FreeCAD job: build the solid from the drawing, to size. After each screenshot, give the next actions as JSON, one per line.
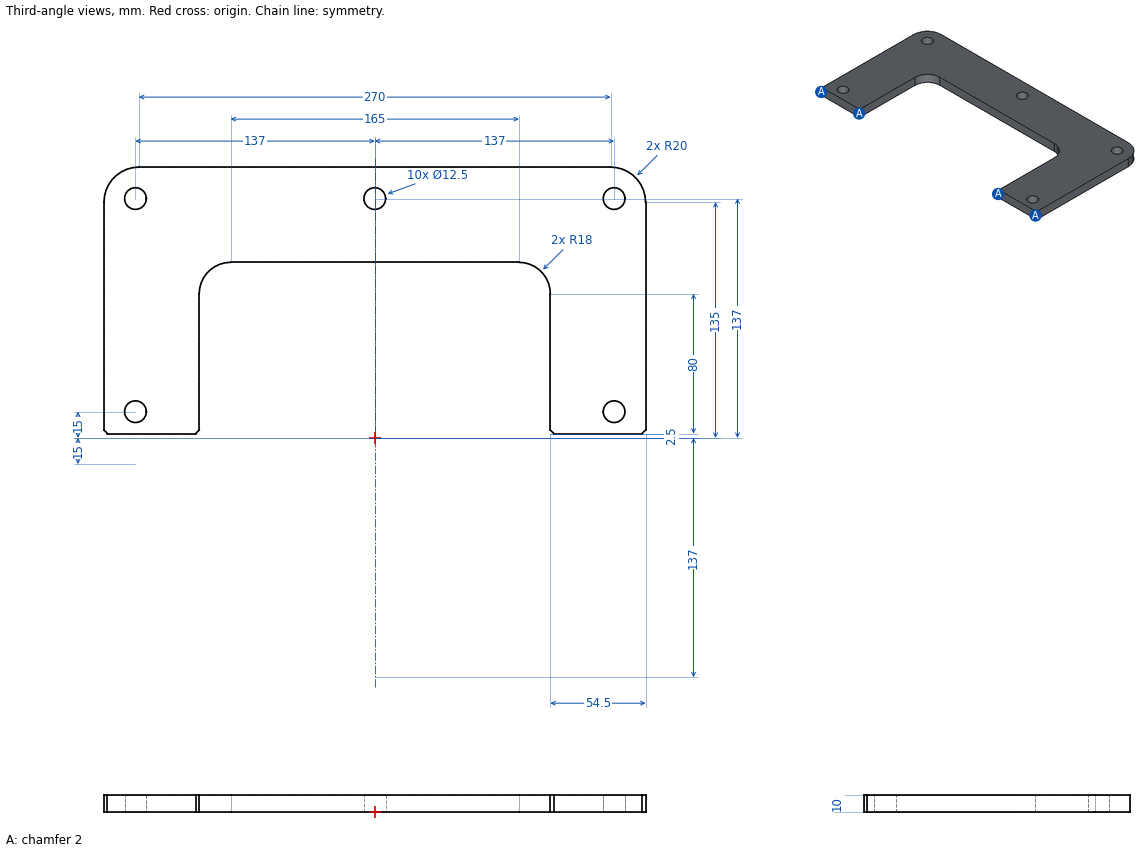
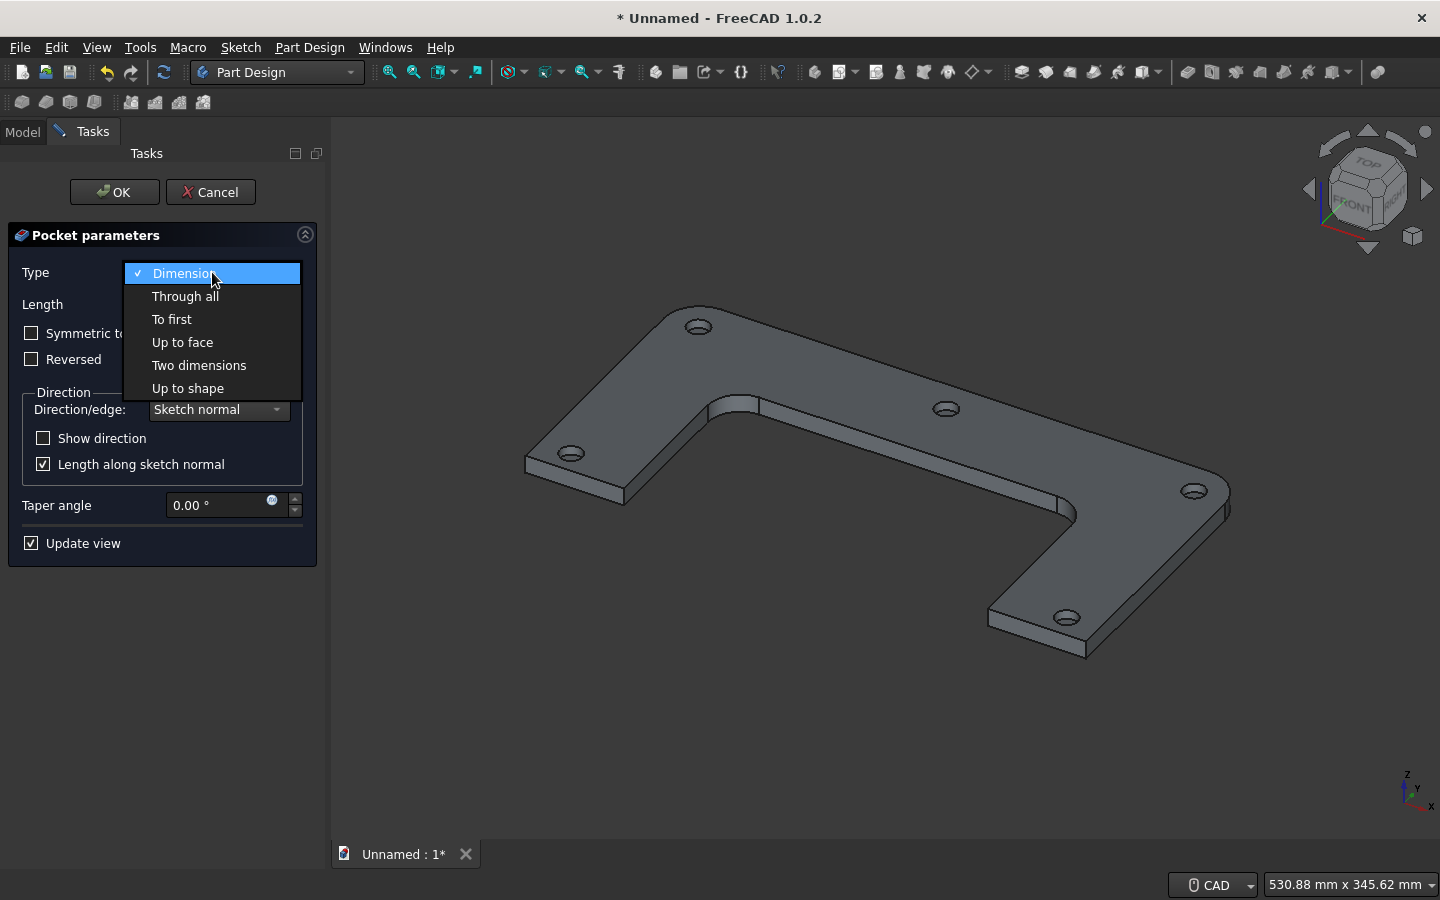
{"action": "left_click", "coordinate": [212, 296]}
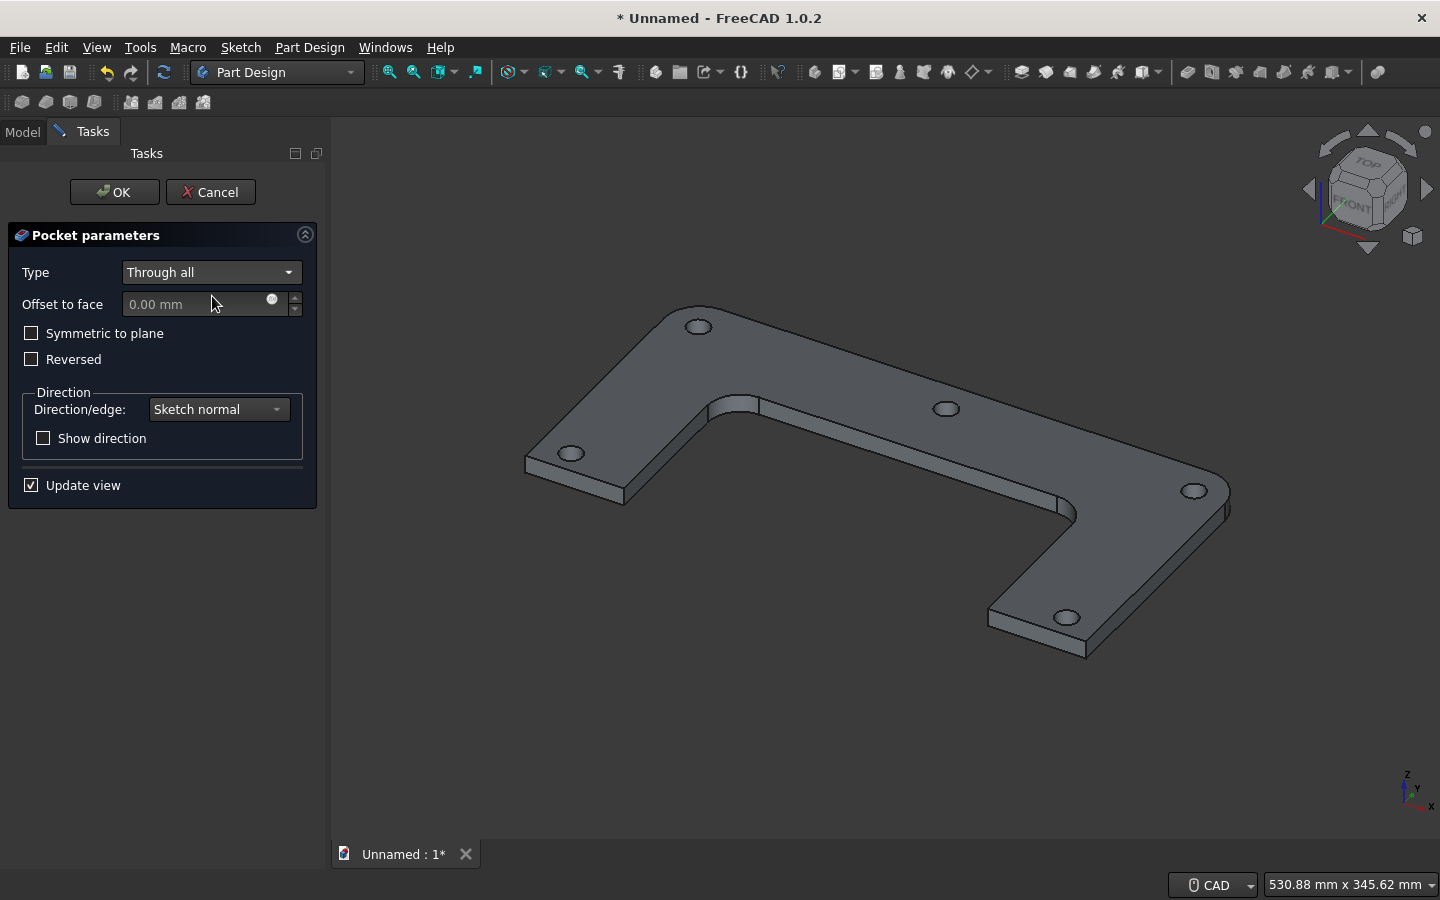
{"action": "left_click", "coordinate": [115, 192]}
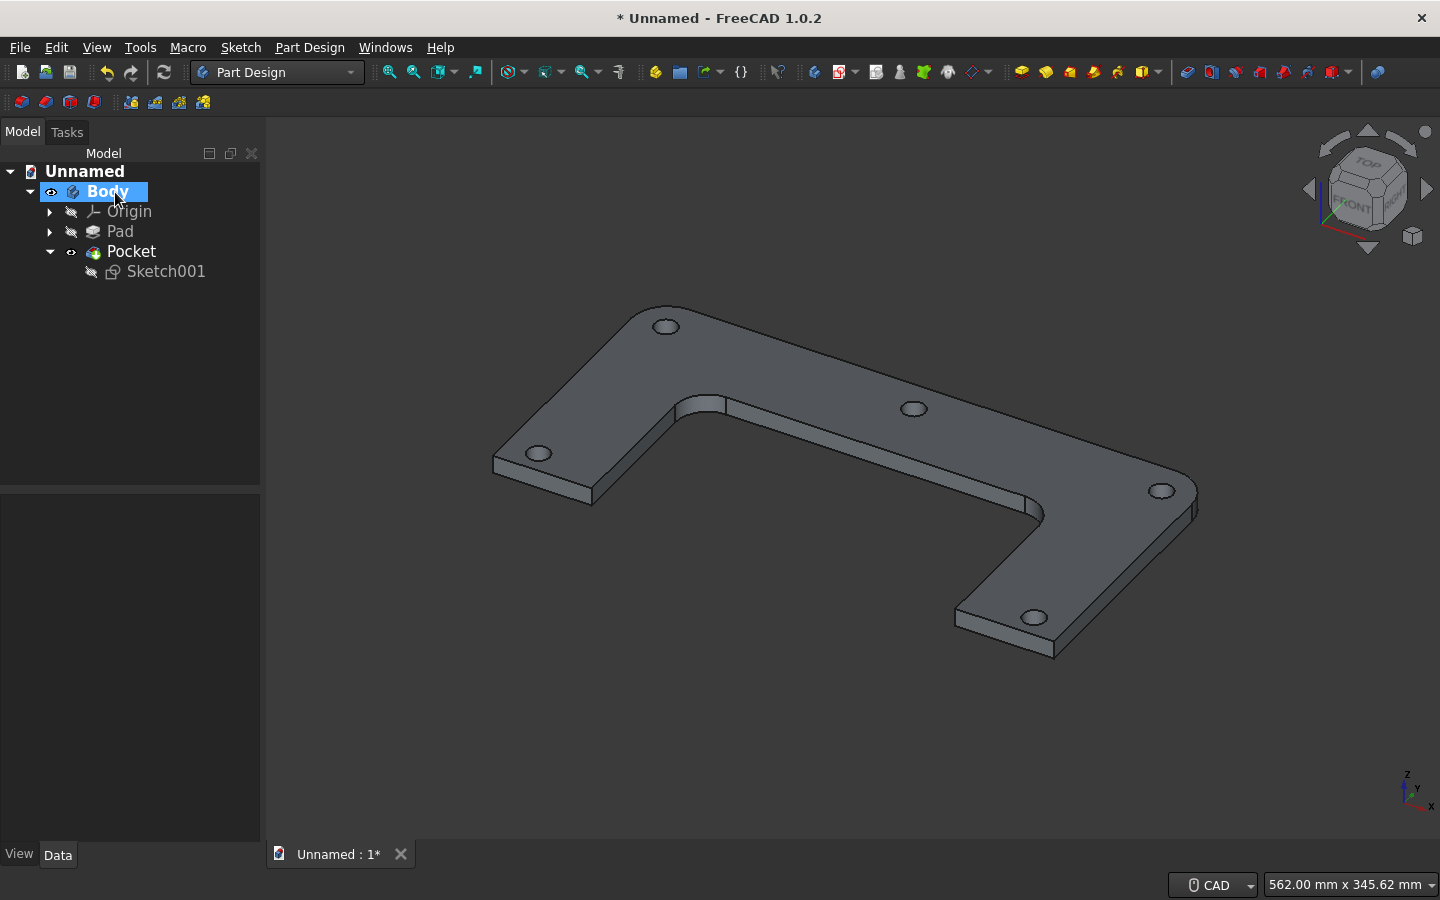
{"action": "left_click", "coordinate": [592, 496]}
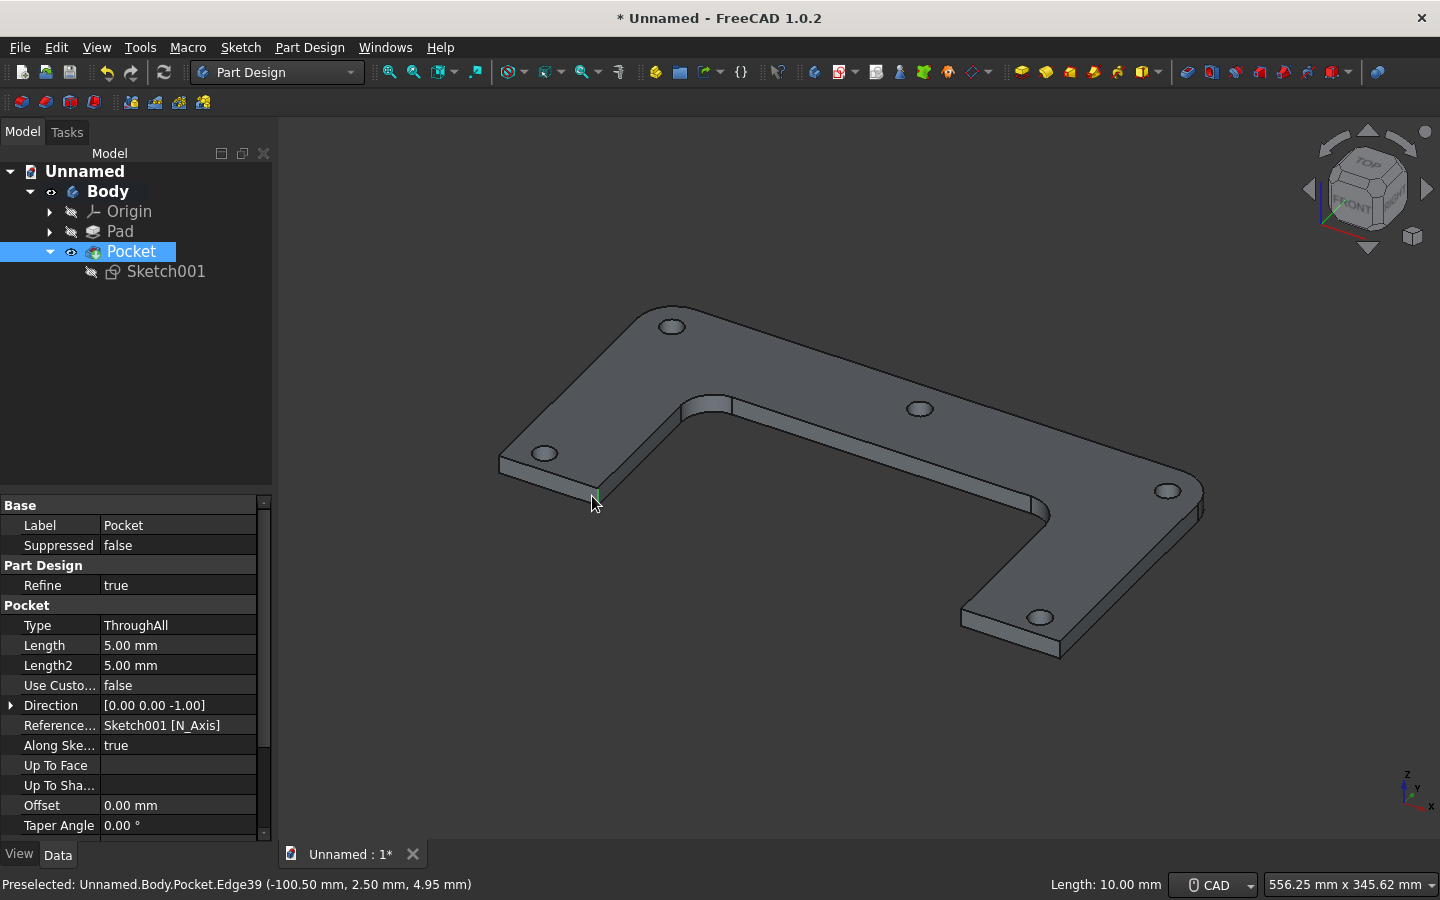
{"action": "left_click", "coordinate": [1060, 649], "text": "ctrl"}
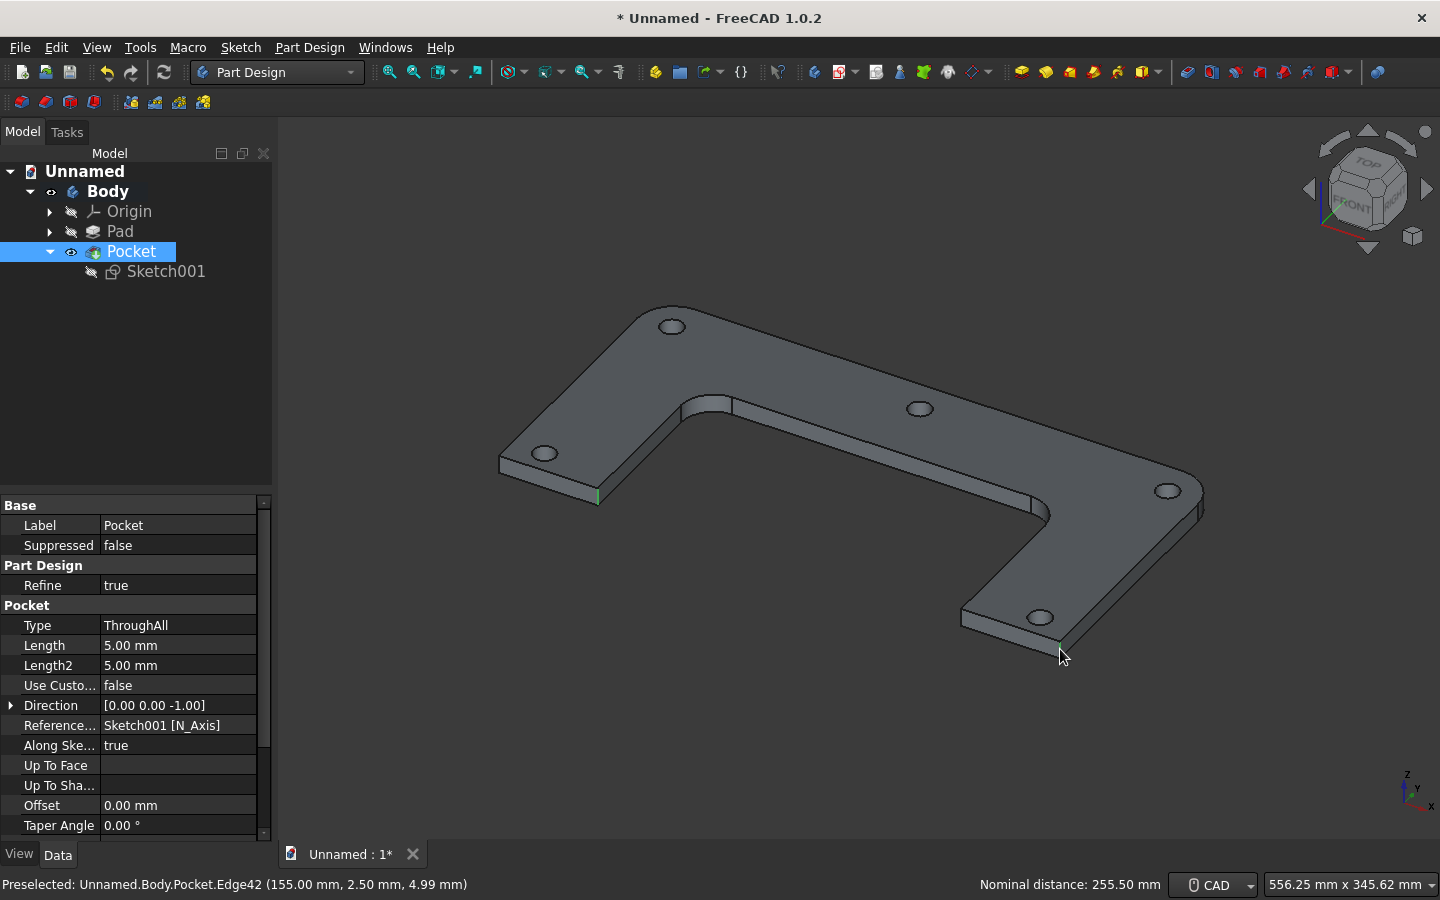
{"action": "scroll", "coordinate": [499, 463], "scroll_direction": "up", "scroll_amount": 4}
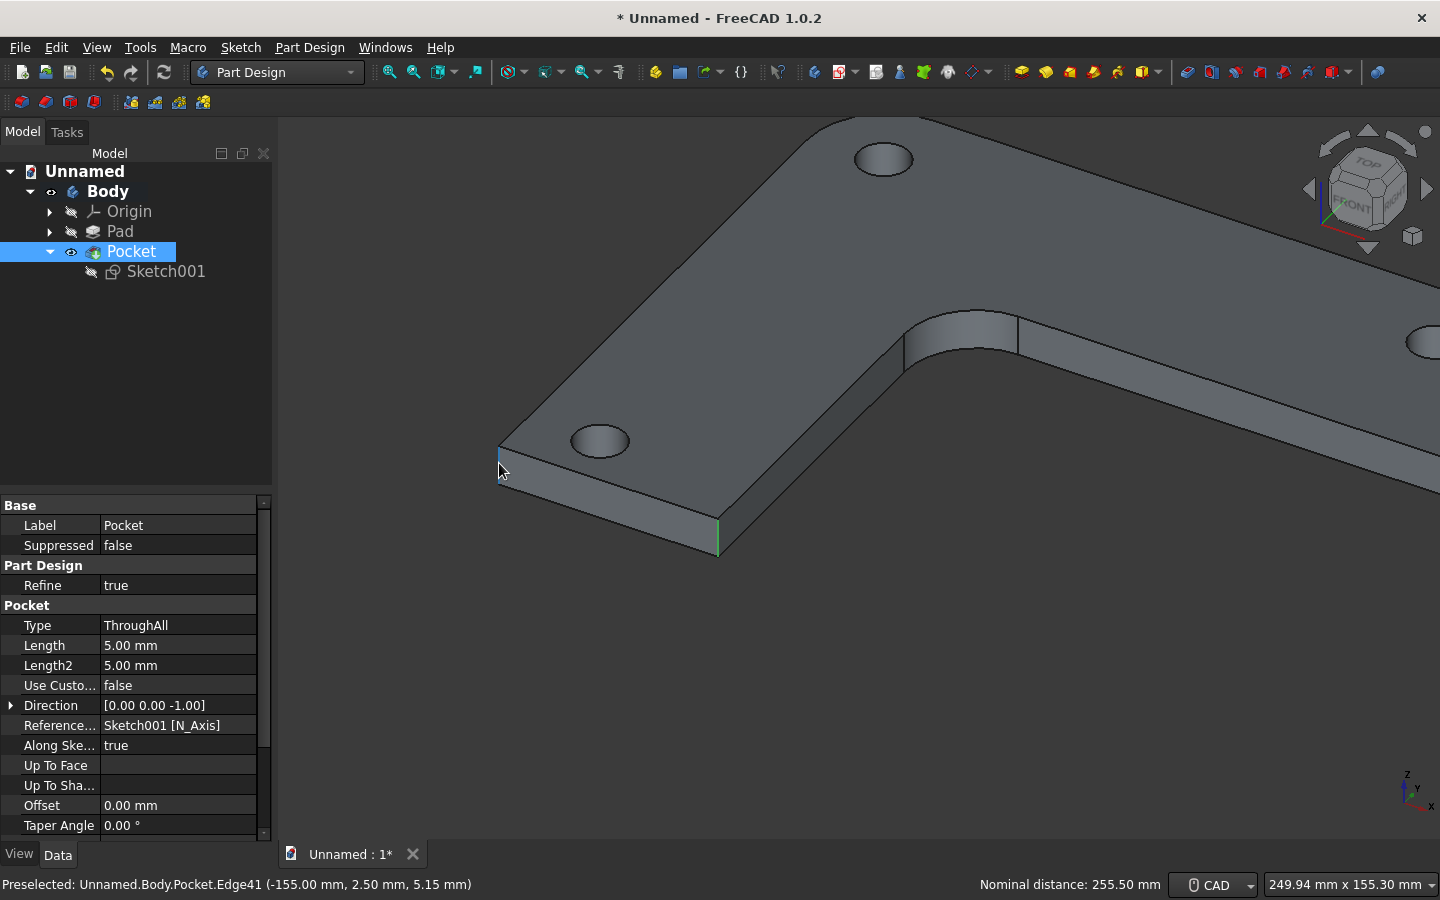
{"action": "key", "text": "v f"}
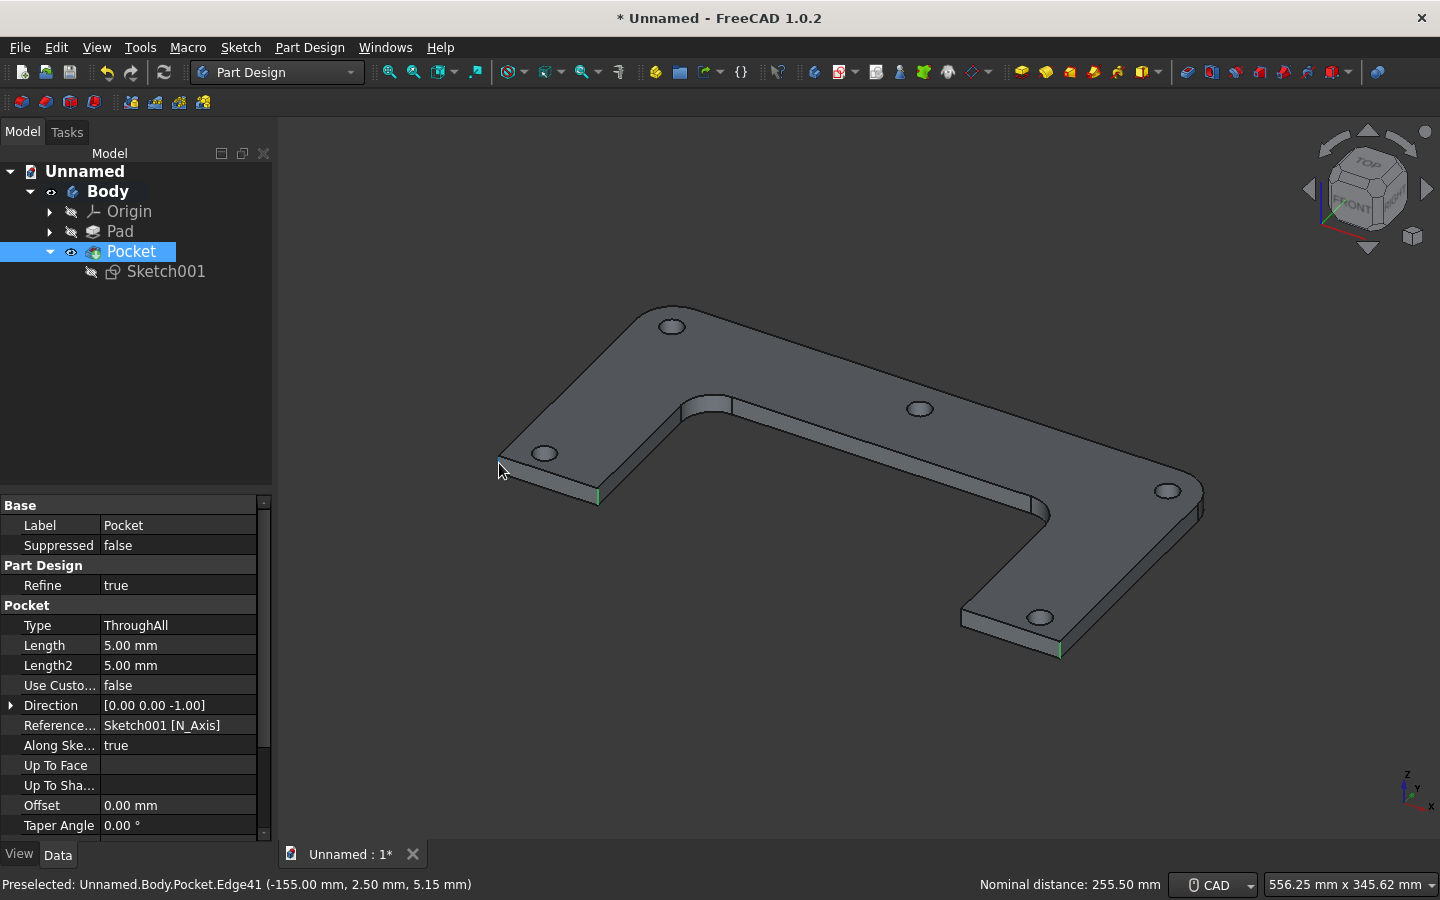
{"action": "key", "text": "0"}